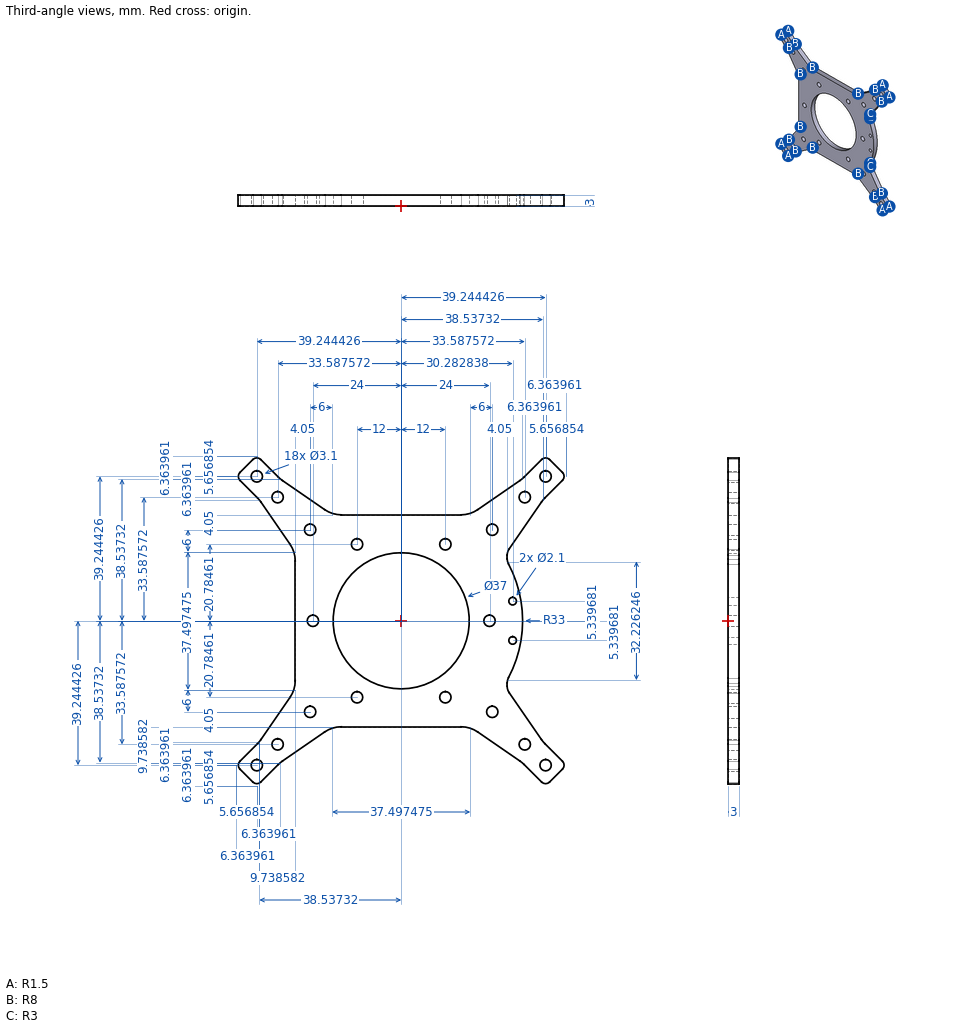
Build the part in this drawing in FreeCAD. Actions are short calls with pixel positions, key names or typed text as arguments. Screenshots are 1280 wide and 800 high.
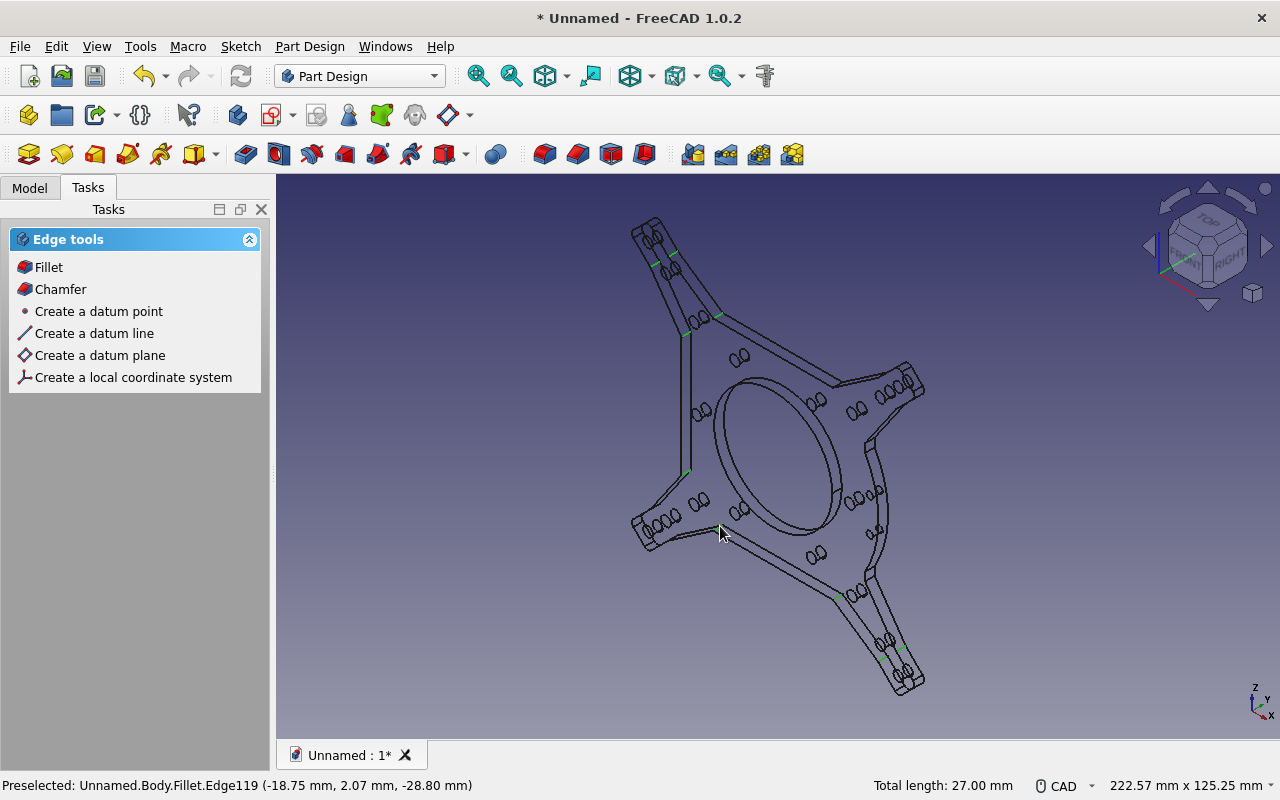
scroll(901, 405, up, 6)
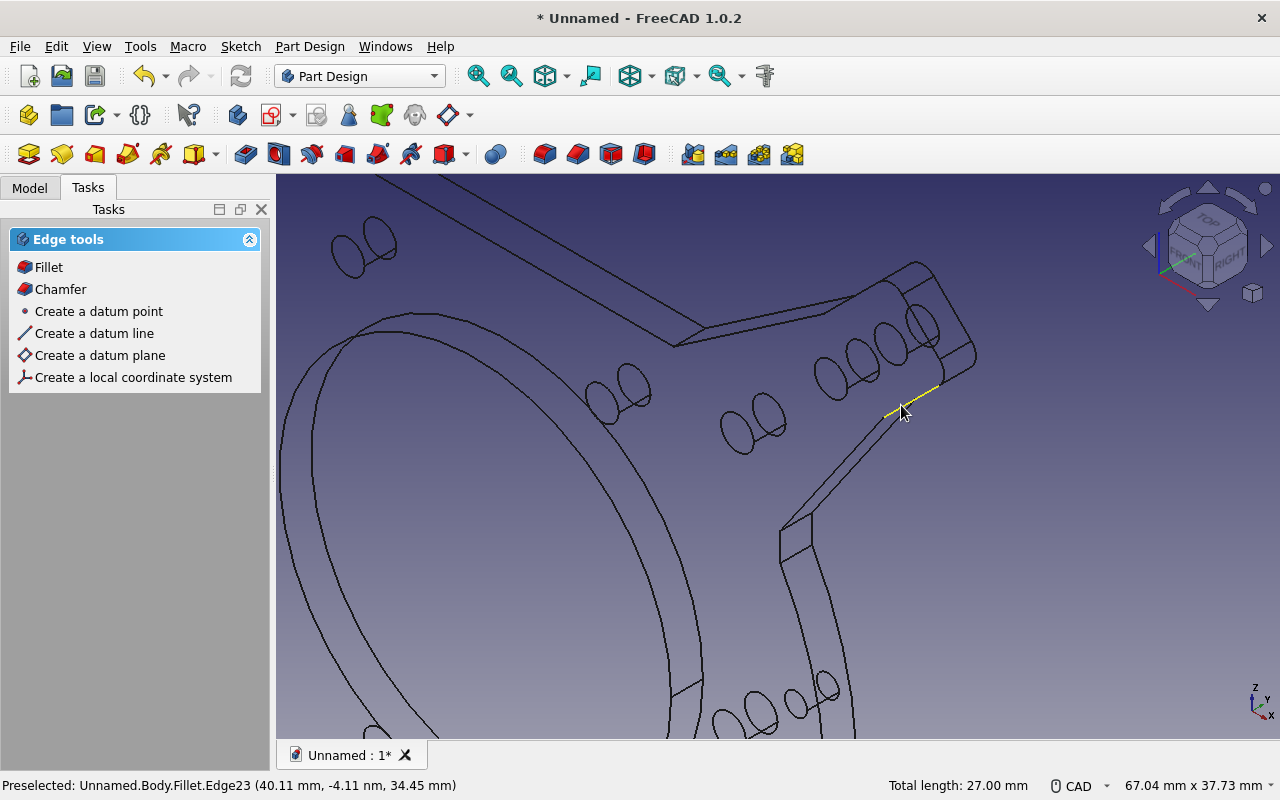
click(693, 335, ctrl)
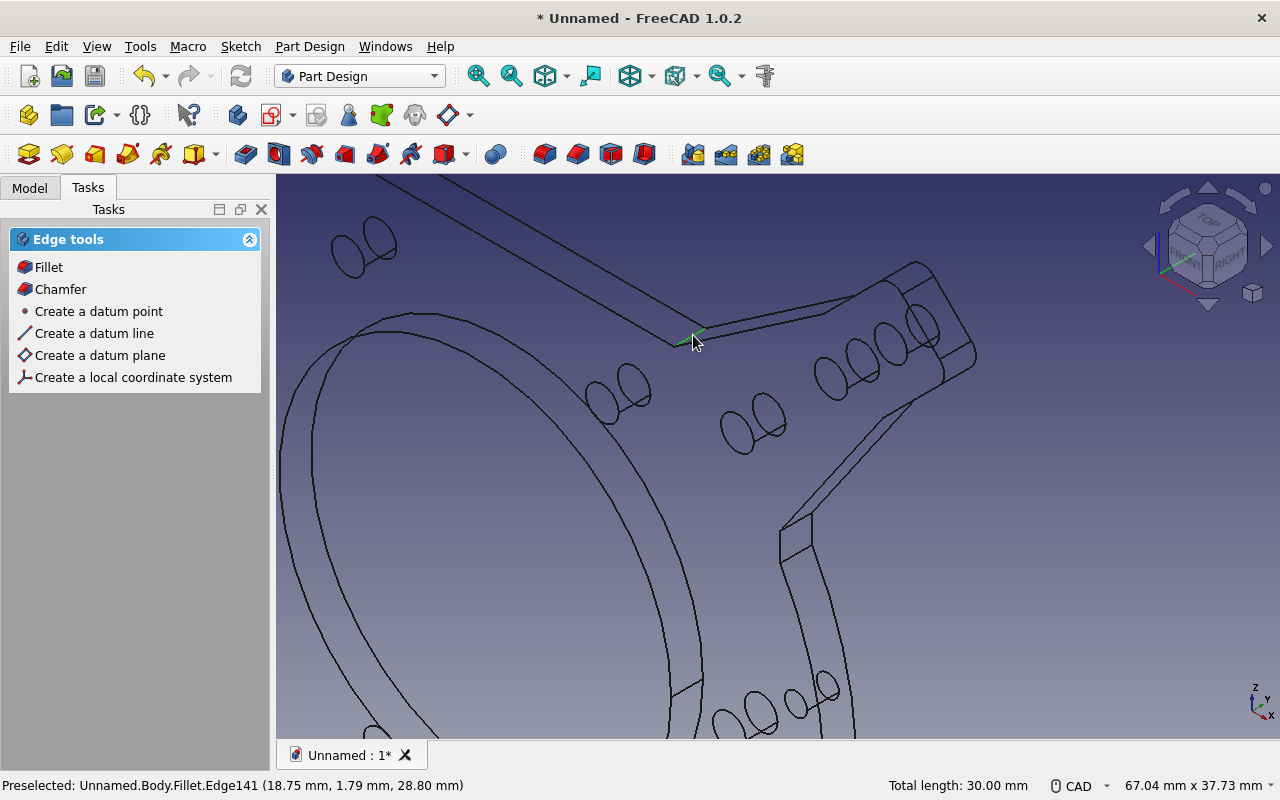
click(479, 76)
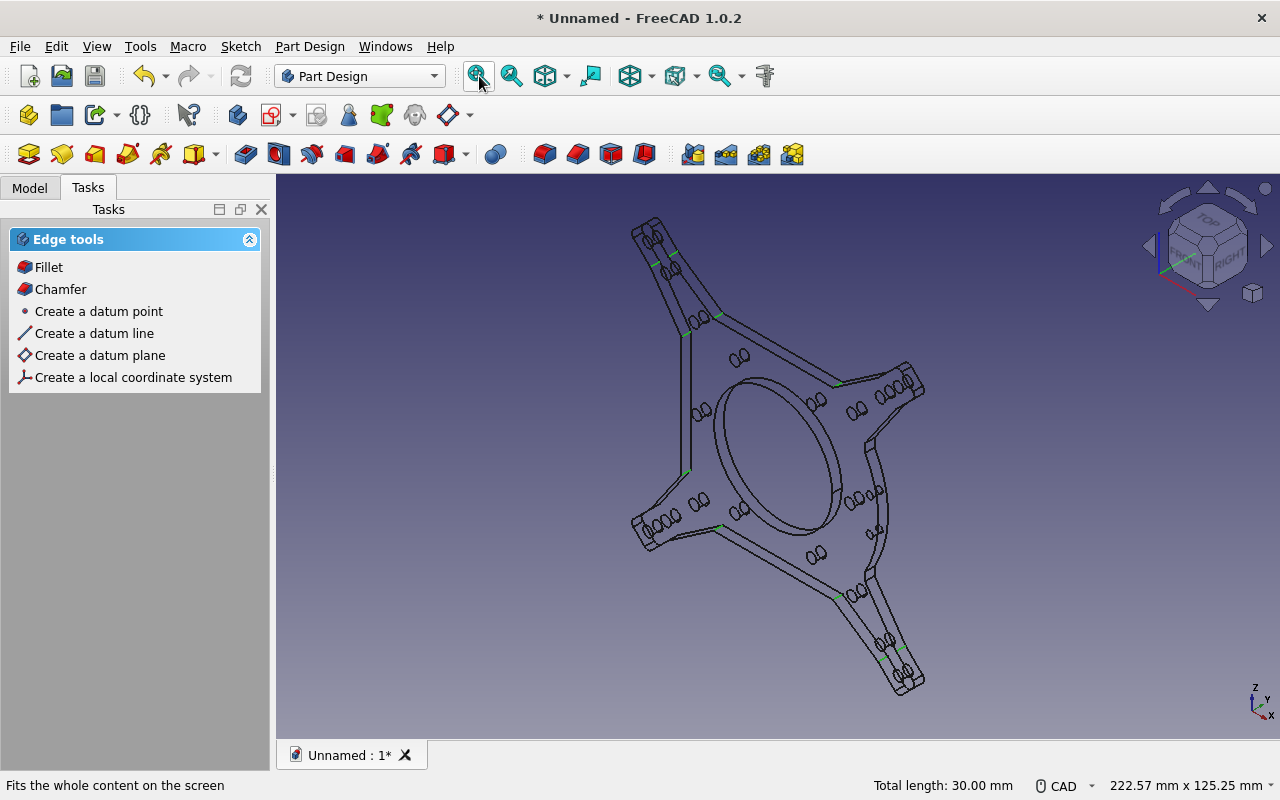
key(2)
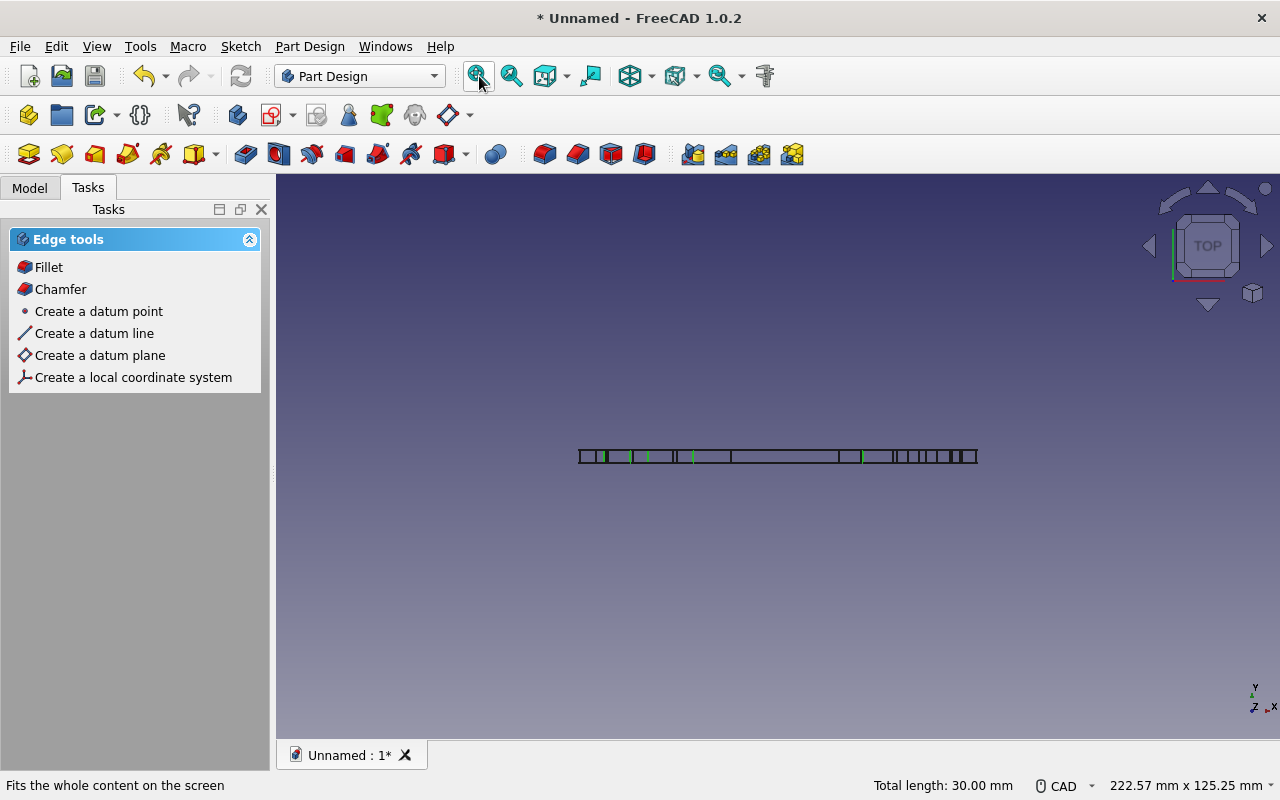
click(479, 76)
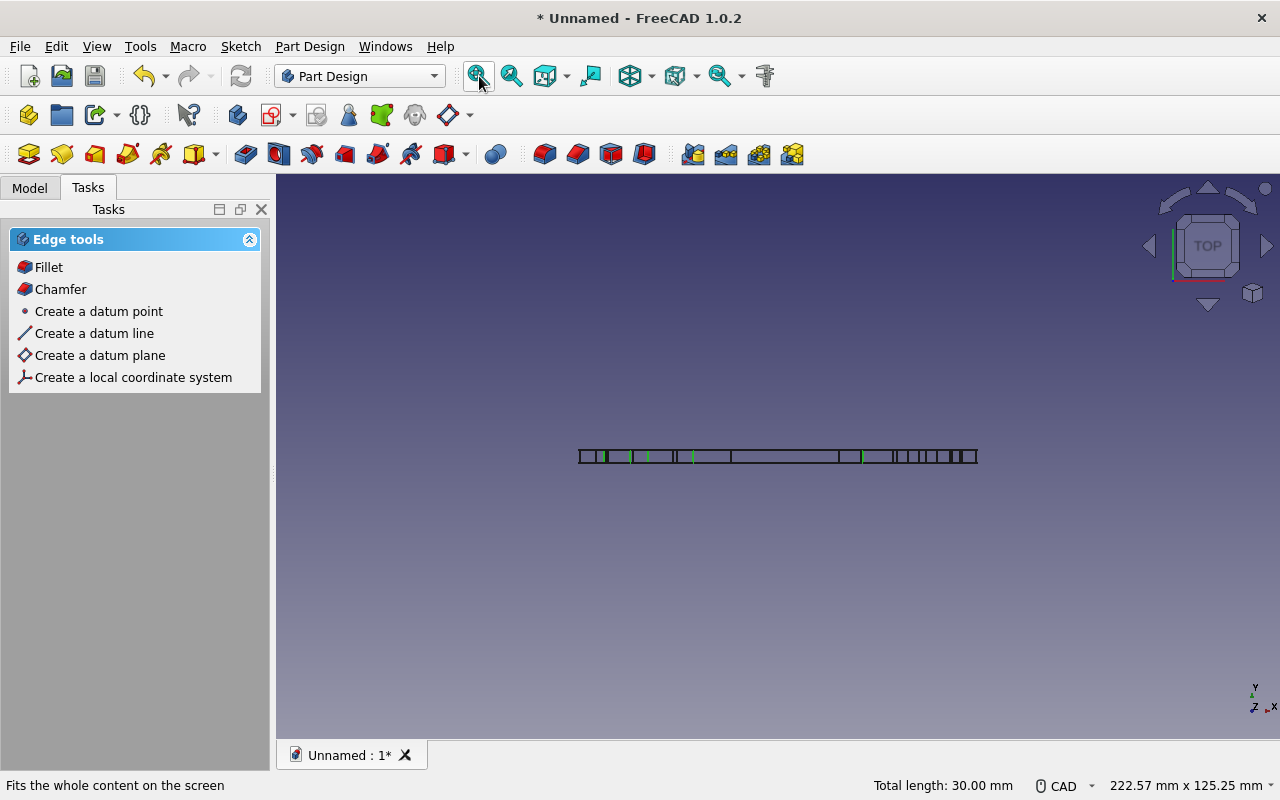
click(926, 455, ctrl)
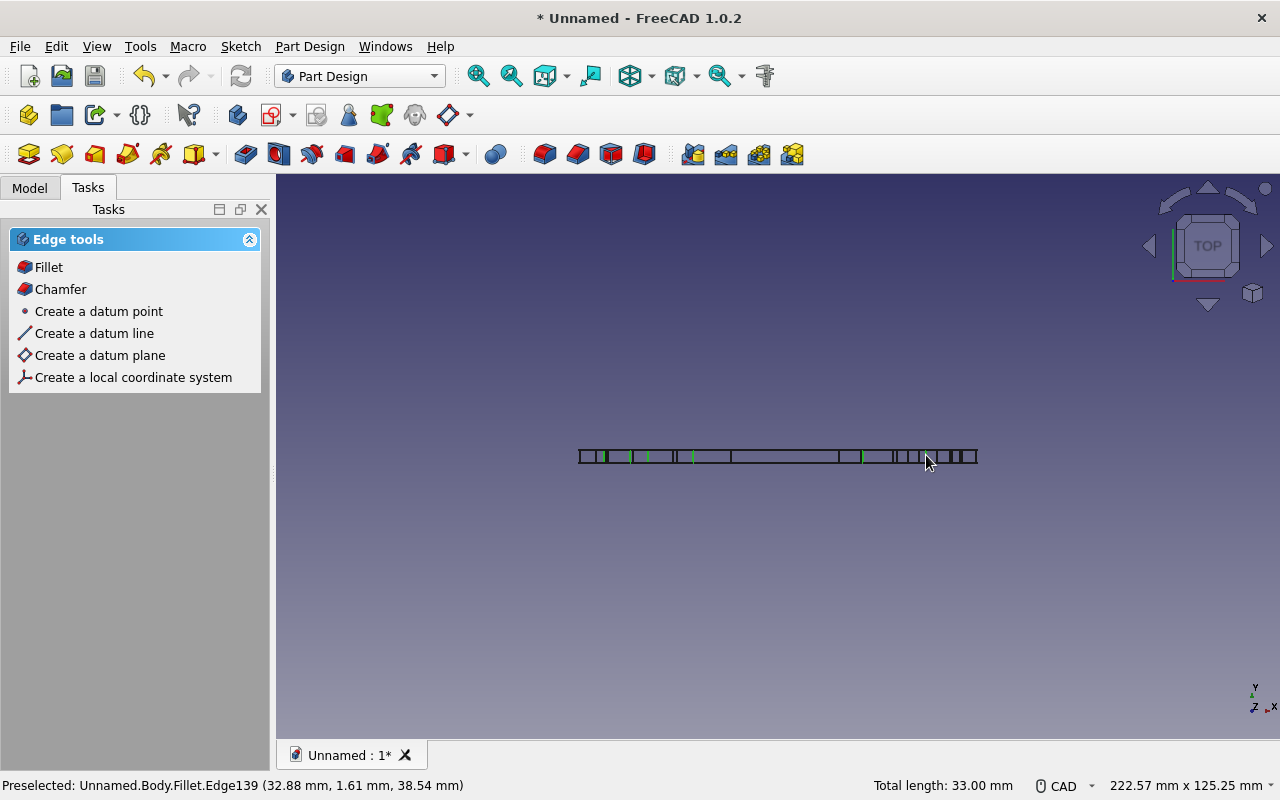
scroll(952, 455, up, 6)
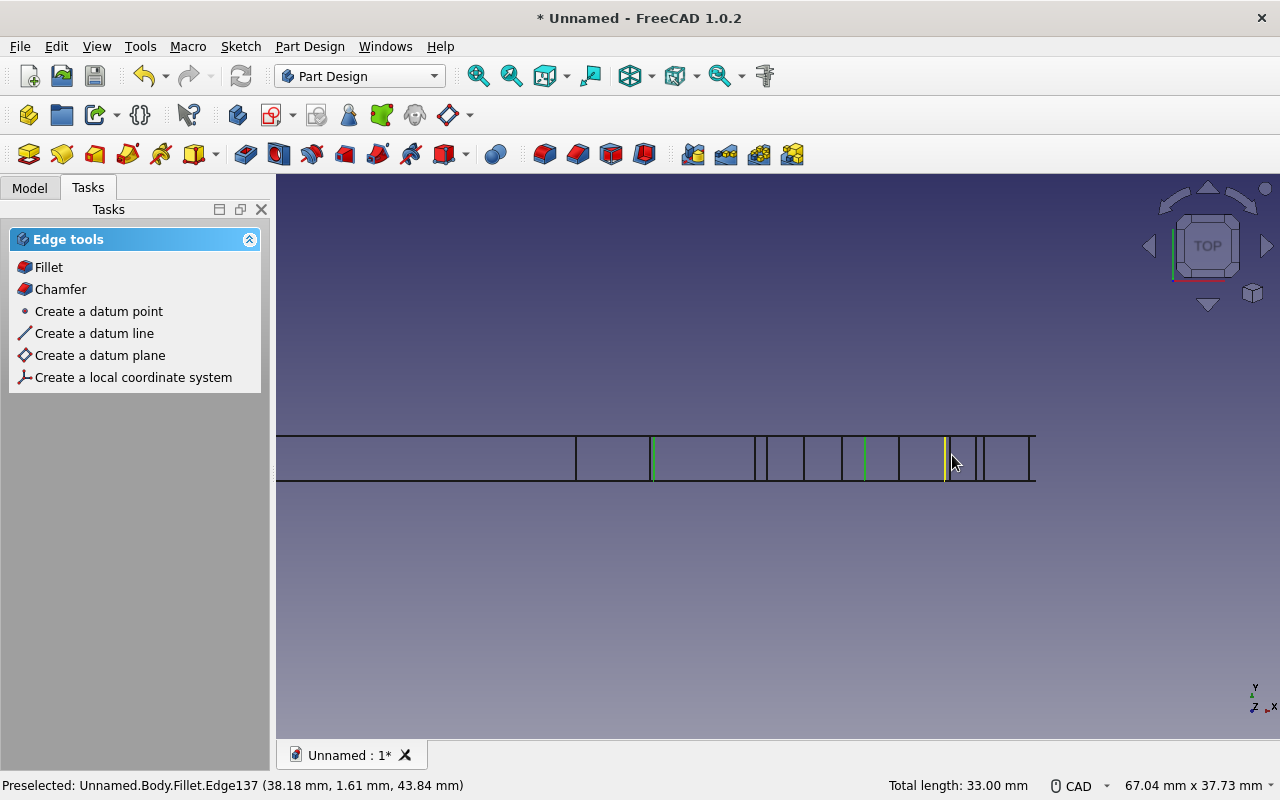
click(479, 76)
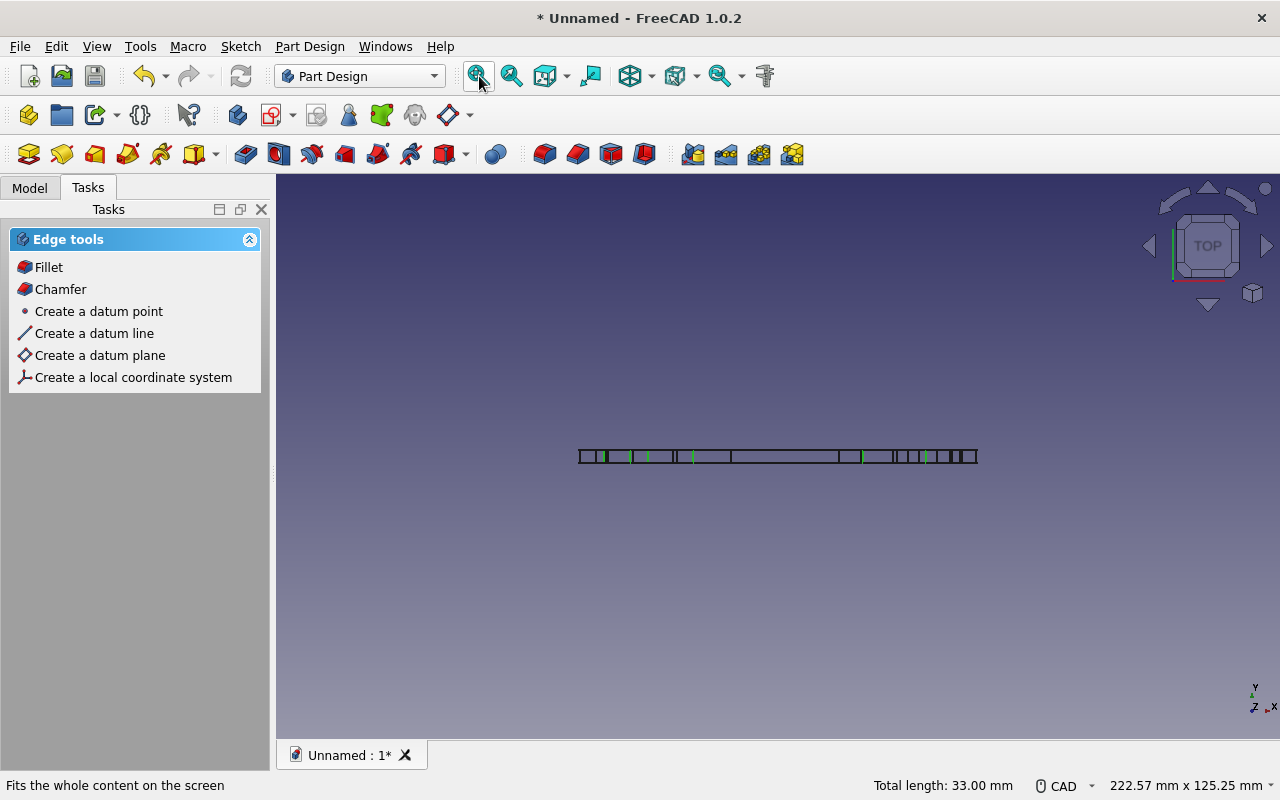
key(1)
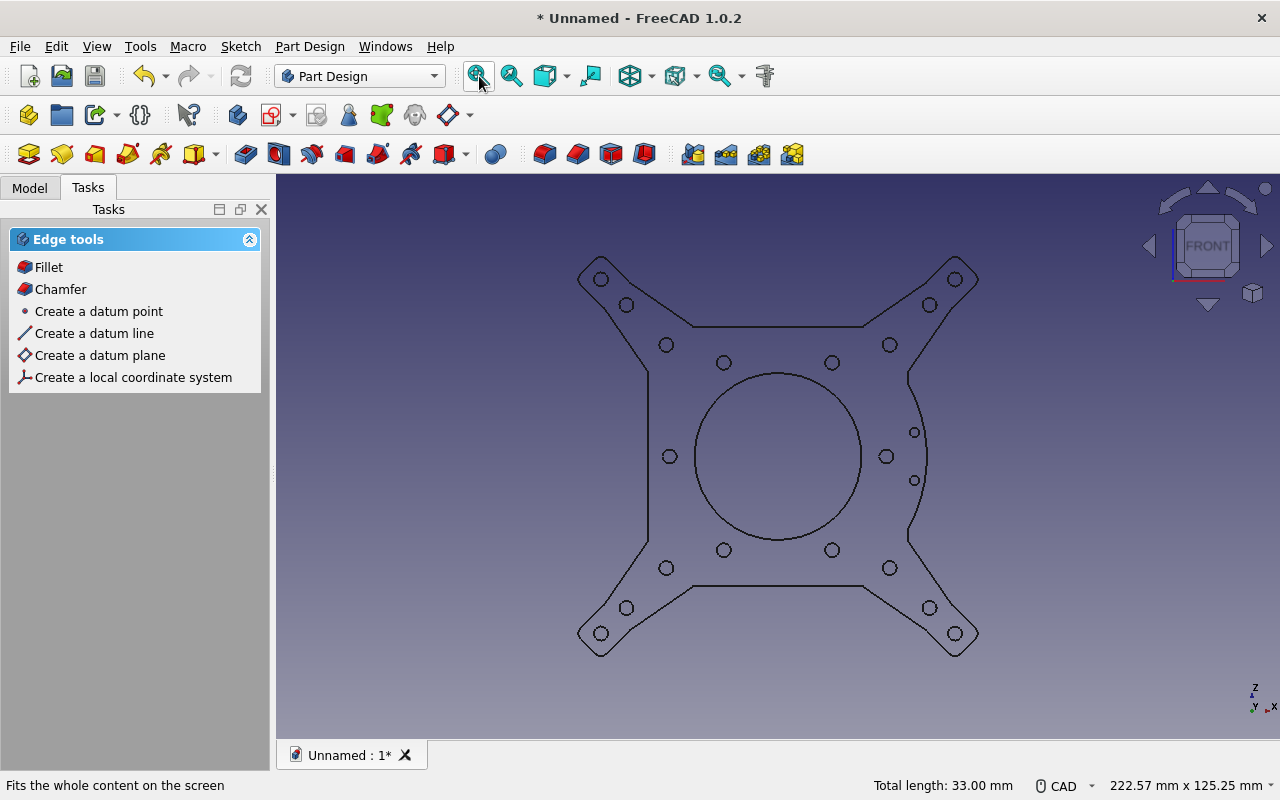
scroll(952, 307, up, 6)